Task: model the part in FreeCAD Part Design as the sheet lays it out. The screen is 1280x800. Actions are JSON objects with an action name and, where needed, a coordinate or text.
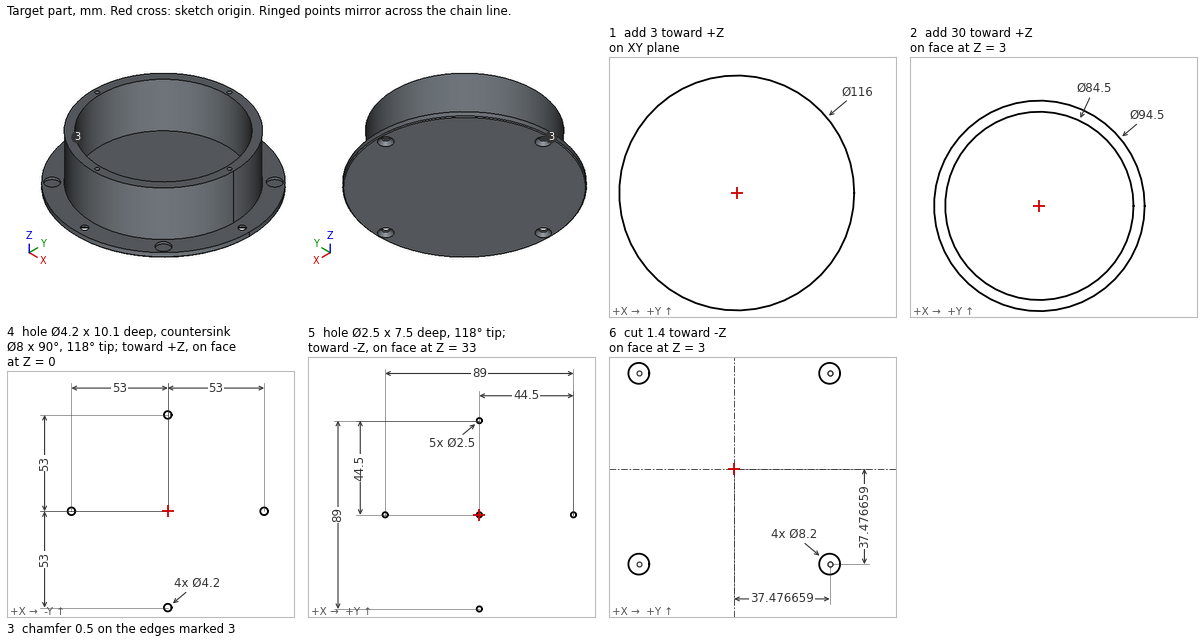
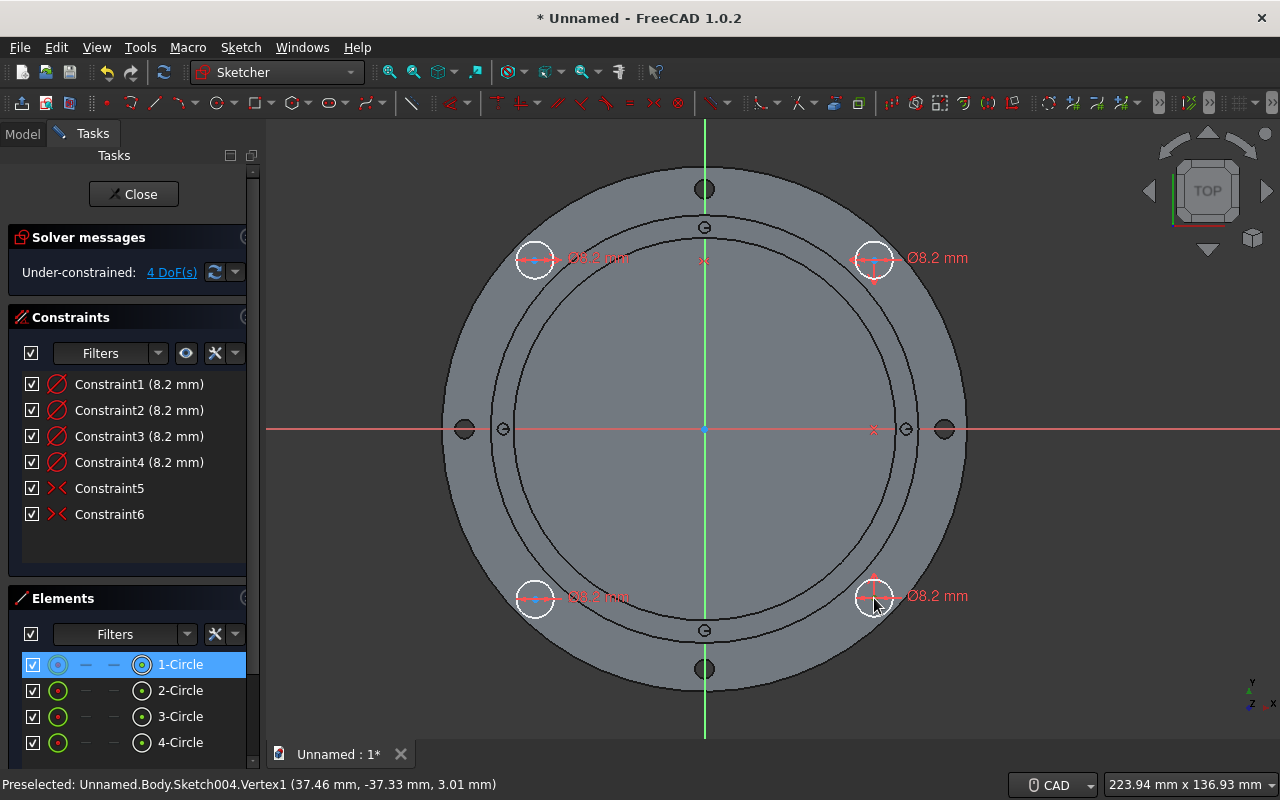
{"action": "left_click", "coordinate": [535, 599]}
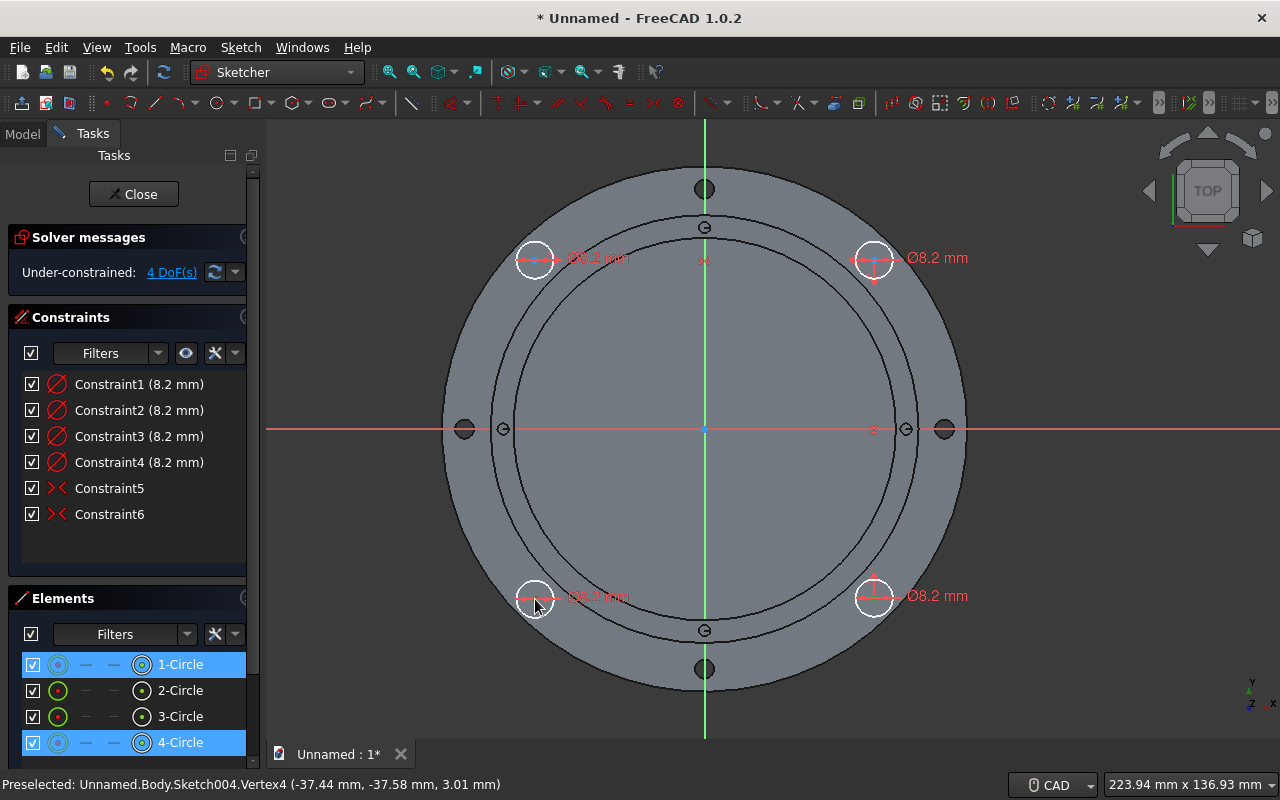
{"action": "left_click", "coordinate": [705, 671]}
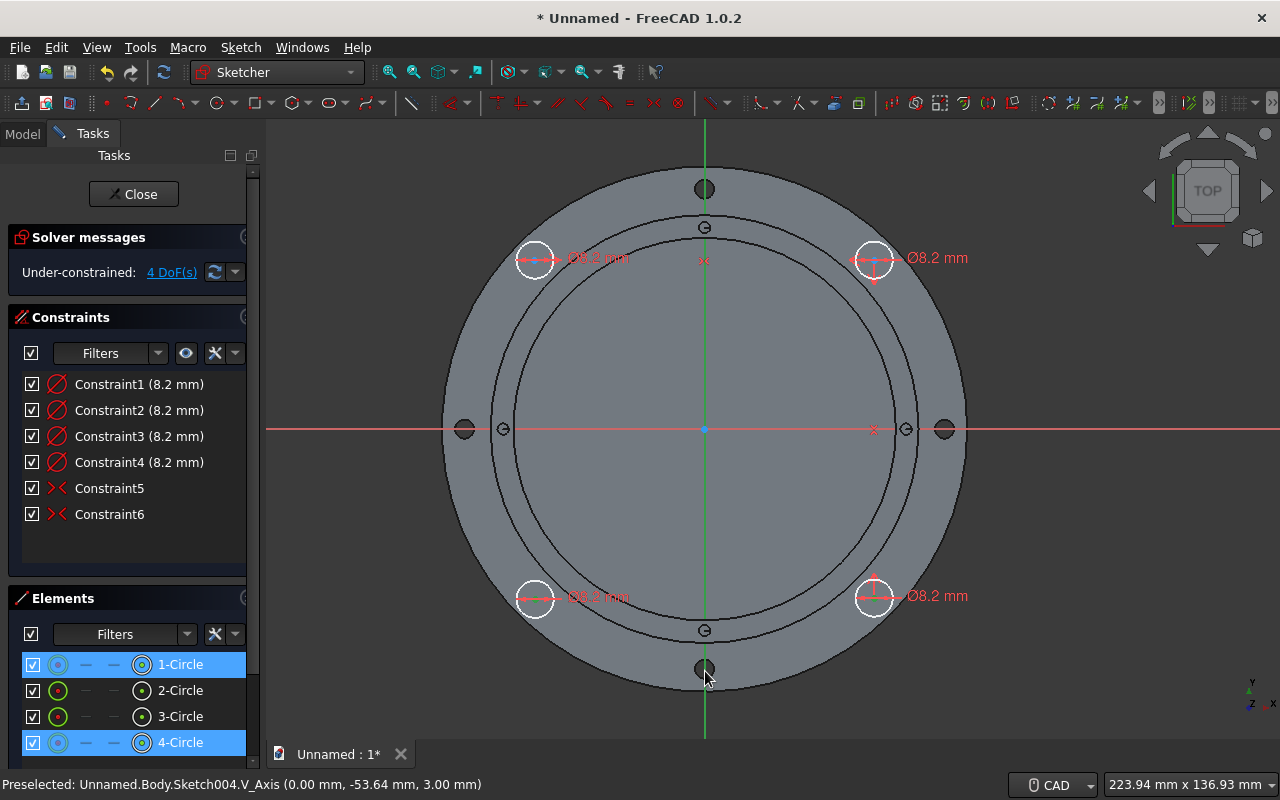
{"action": "left_click", "coordinate": [654, 104]}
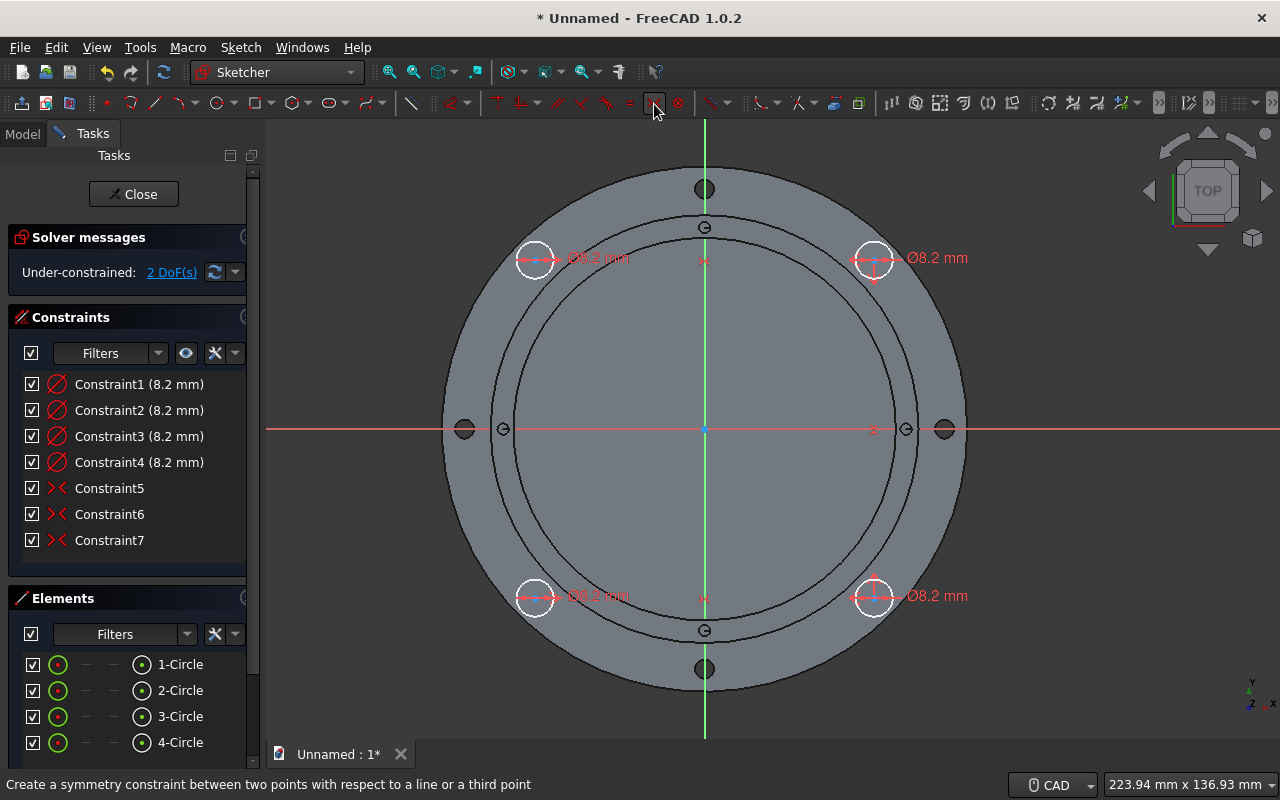
{"action": "left_click", "coordinate": [450, 104]}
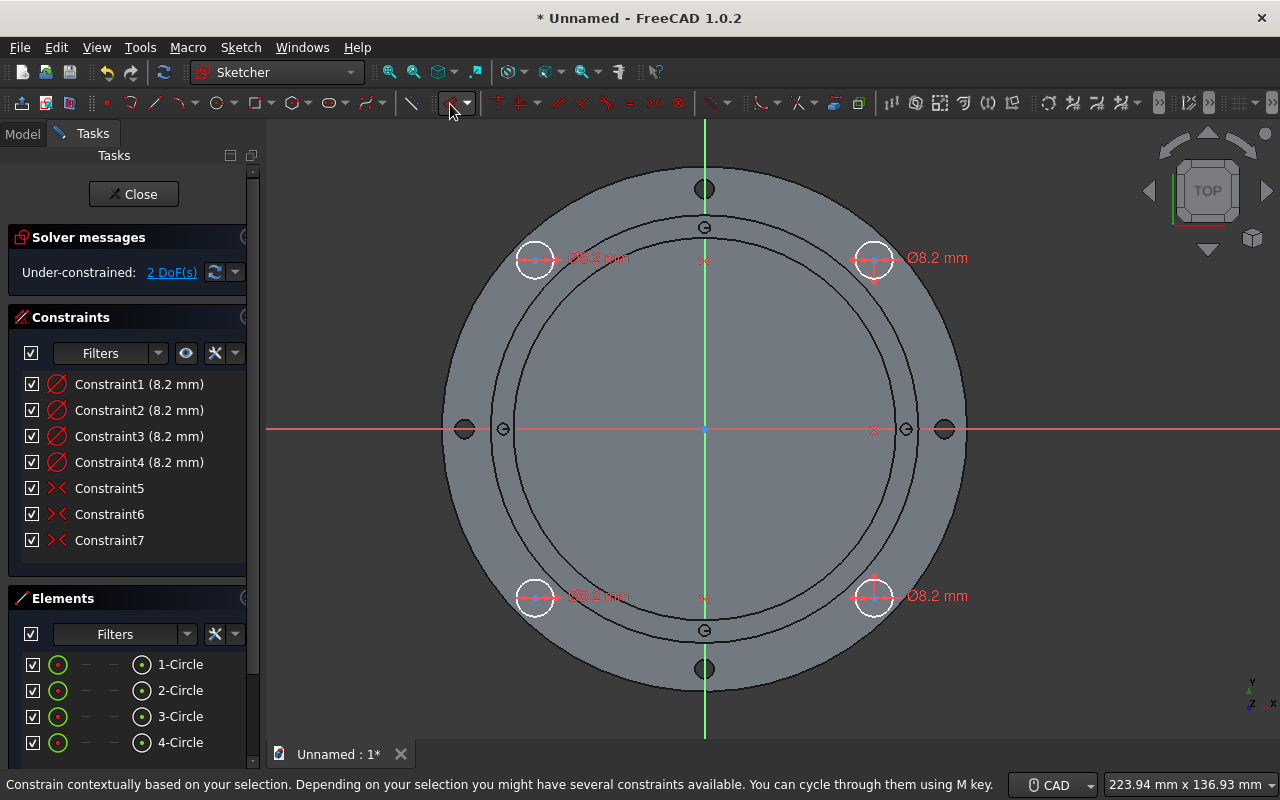
{"action": "left_click", "coordinate": [874, 598]}
{"action": "left_click", "coordinate": [789, 632]}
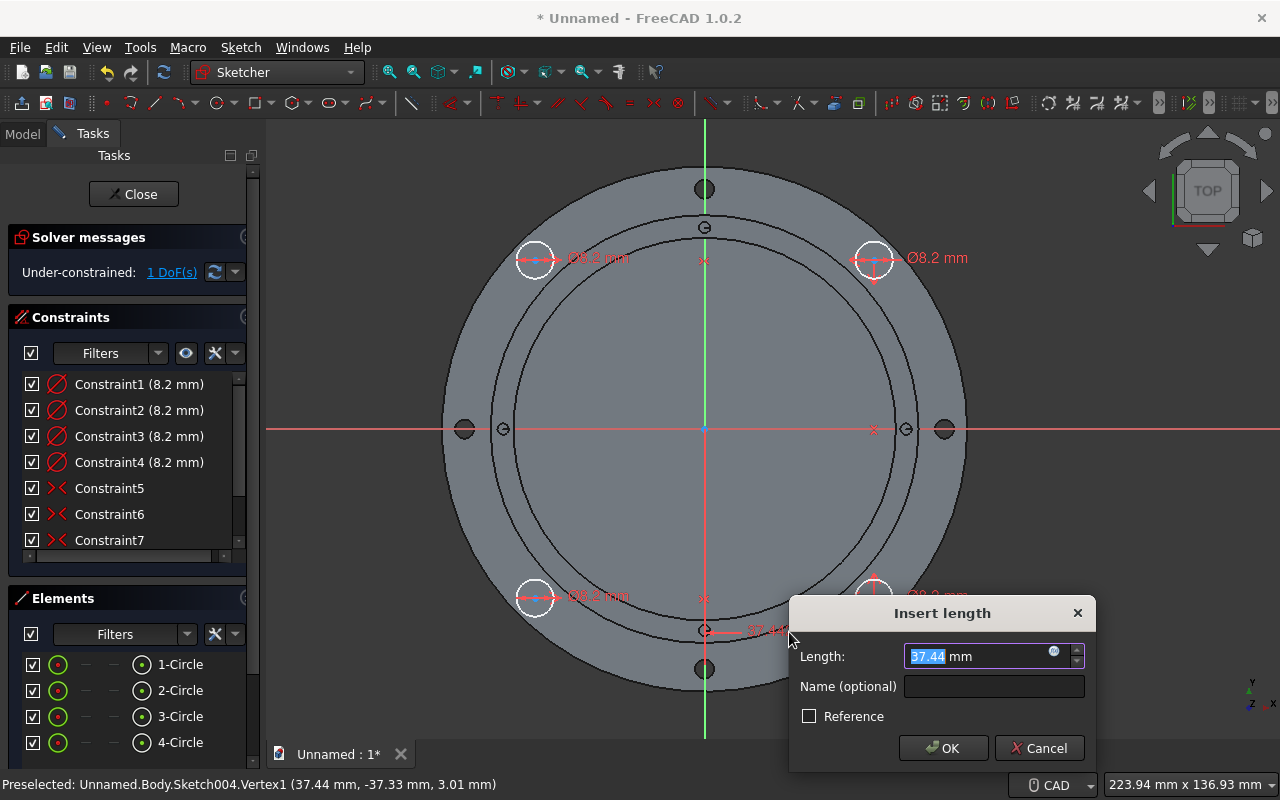
{"action": "type", "text": "37.476659"}
{"action": "key", "text": "Return"}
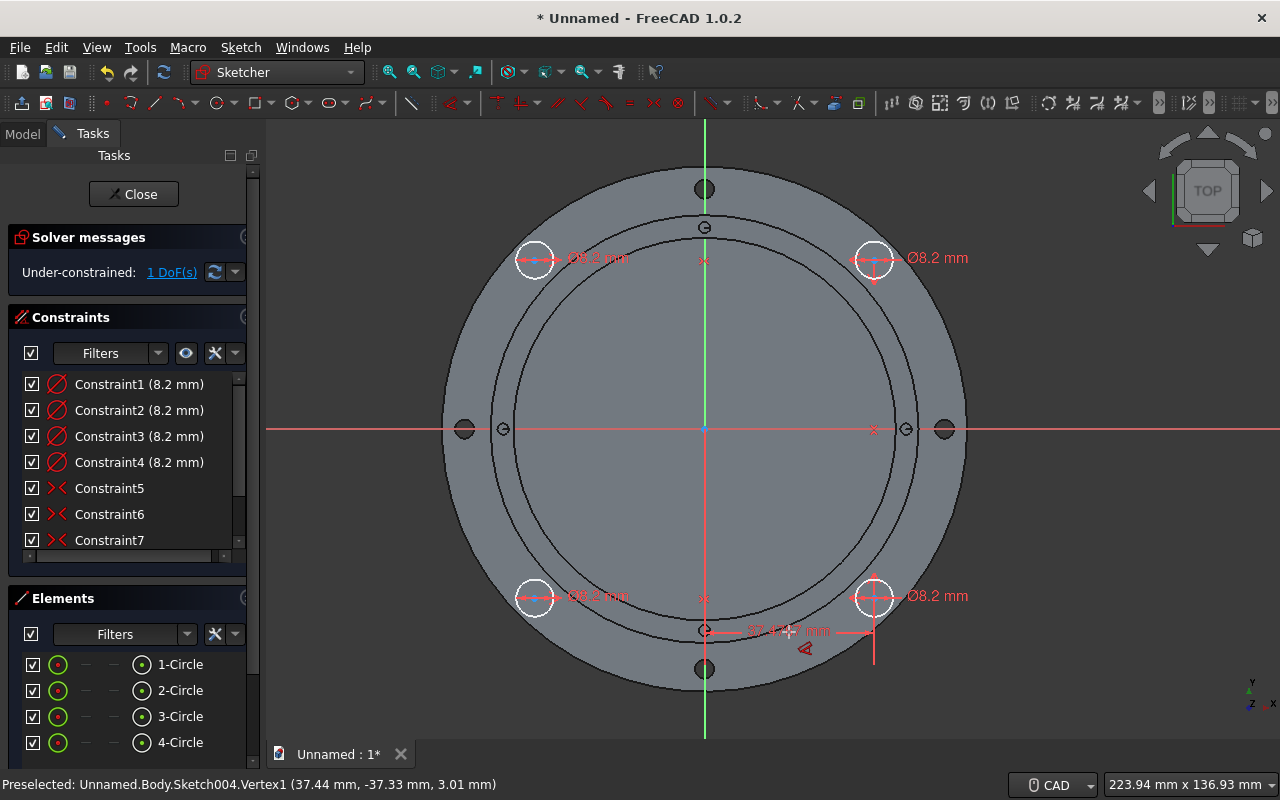
{"action": "left_click", "coordinate": [874, 598]}
{"action": "left_click", "coordinate": [908, 514]}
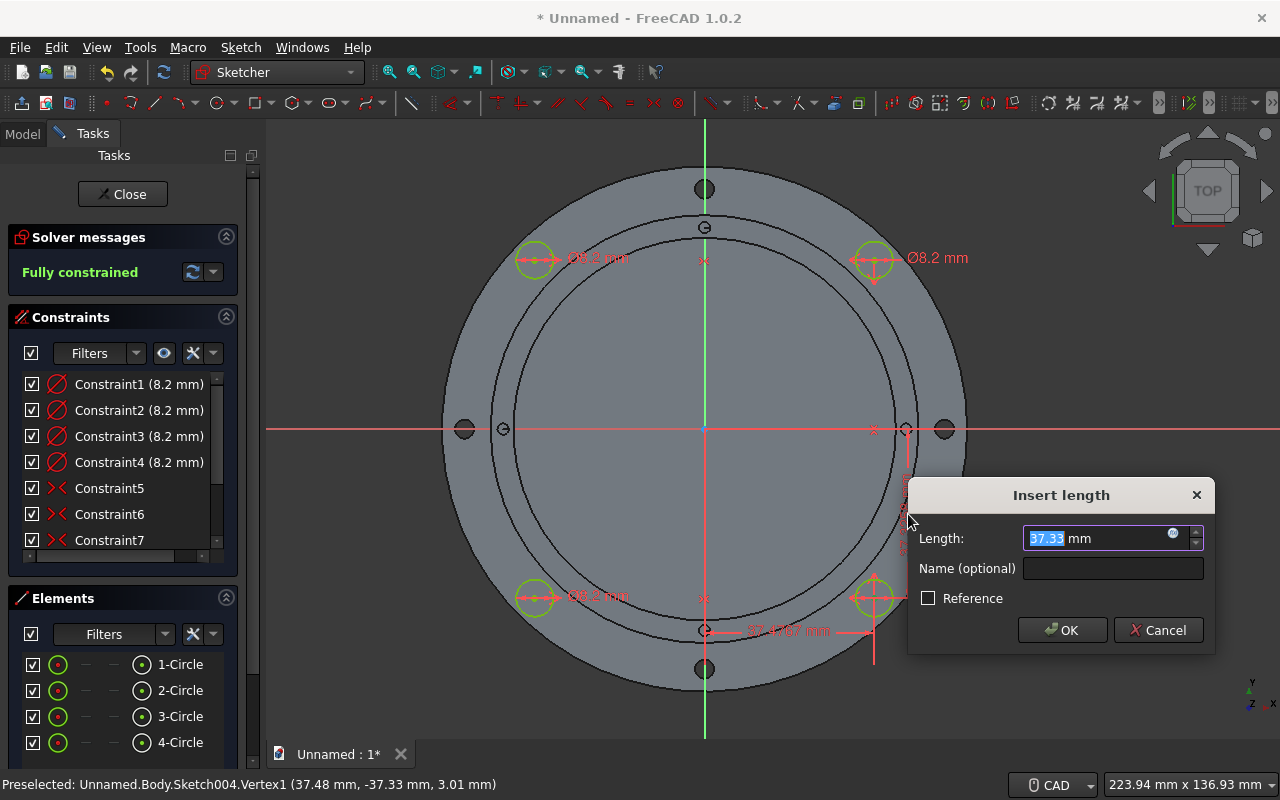
{"action": "type", "text": "37.476659"}
{"action": "key", "text": "Return"}
{"action": "key", "text": "Escape"}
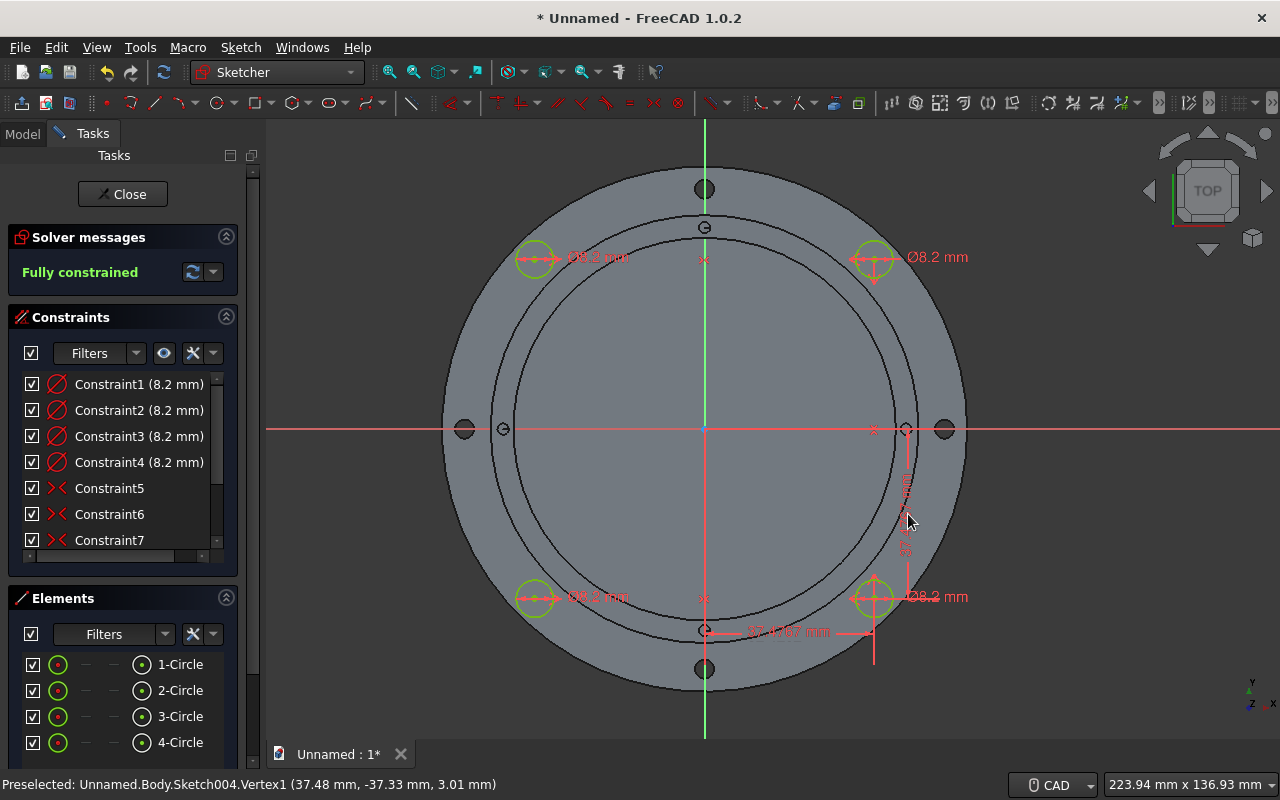
{"action": "left_click", "coordinate": [123, 194]}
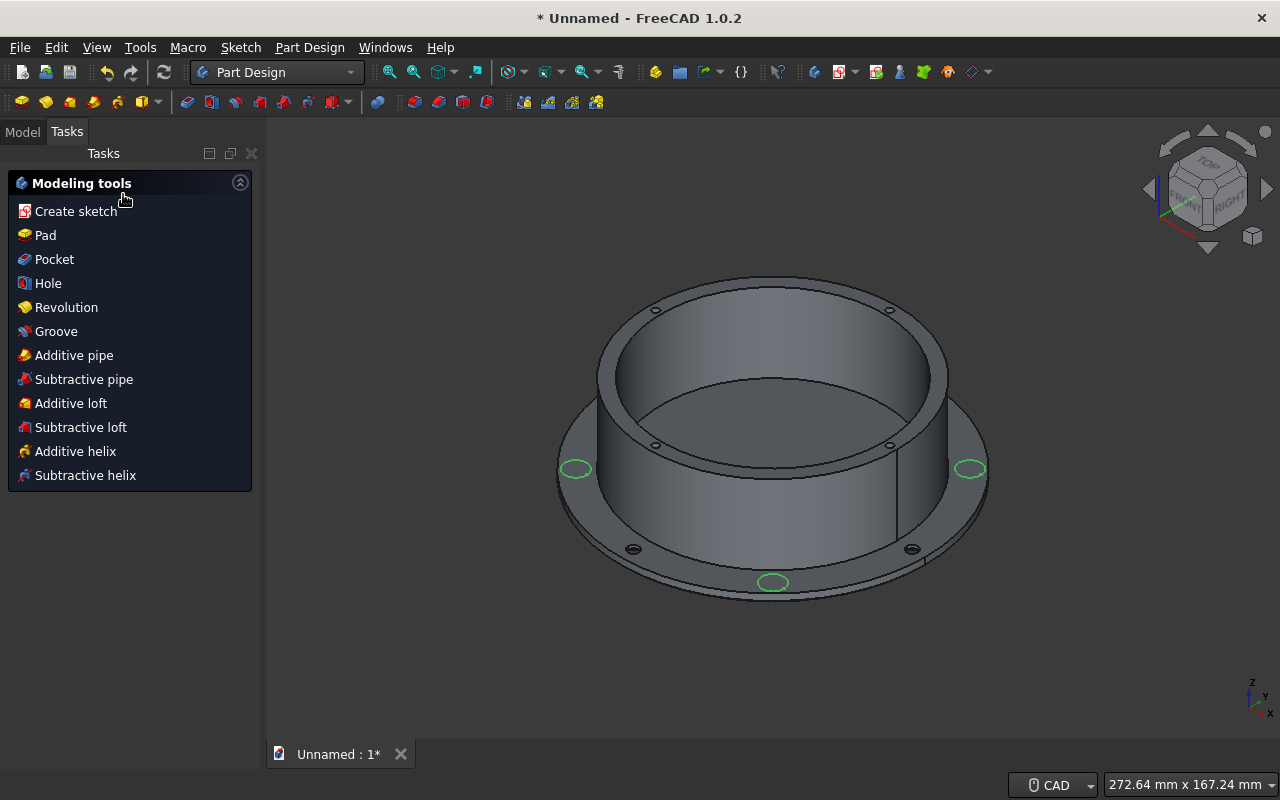
{"action": "left_click", "coordinate": [188, 102]}